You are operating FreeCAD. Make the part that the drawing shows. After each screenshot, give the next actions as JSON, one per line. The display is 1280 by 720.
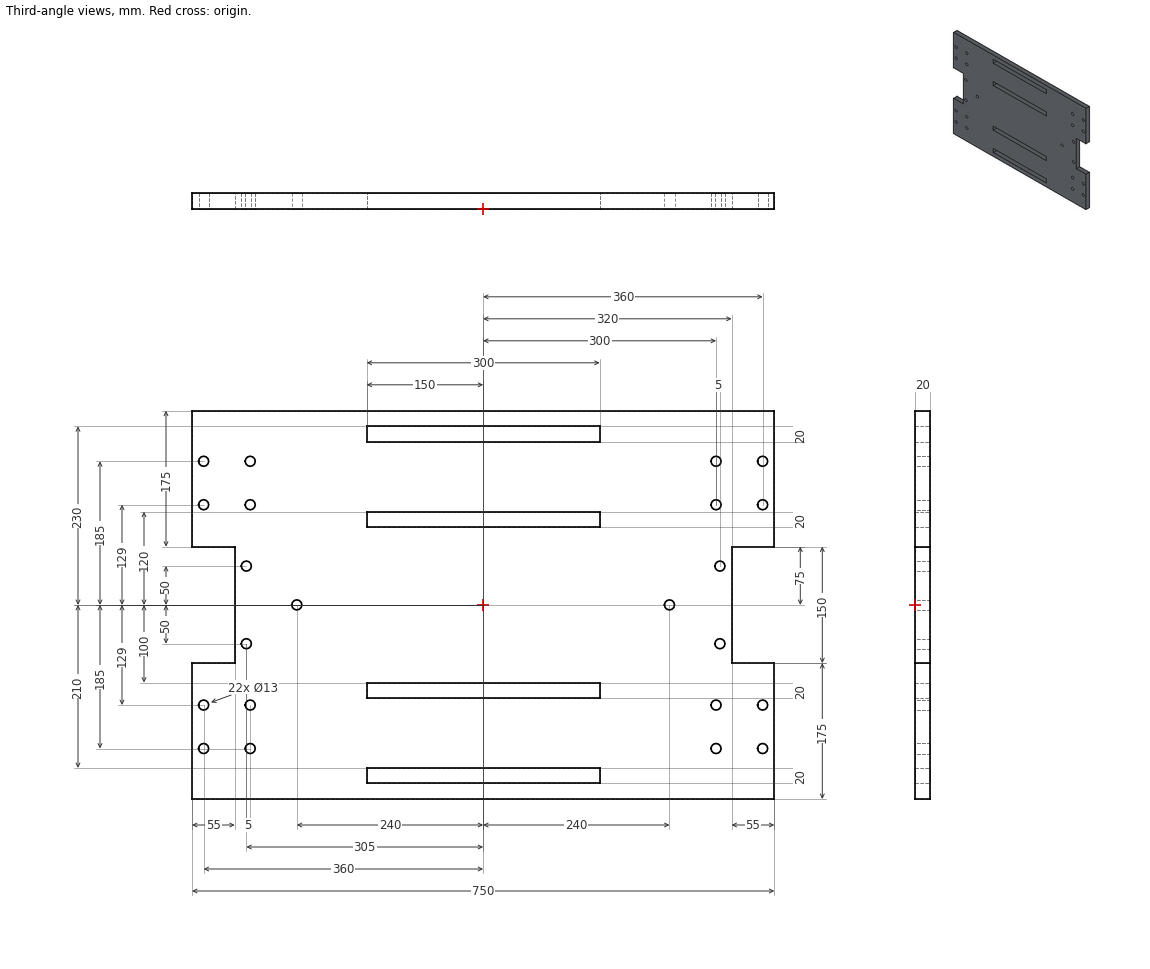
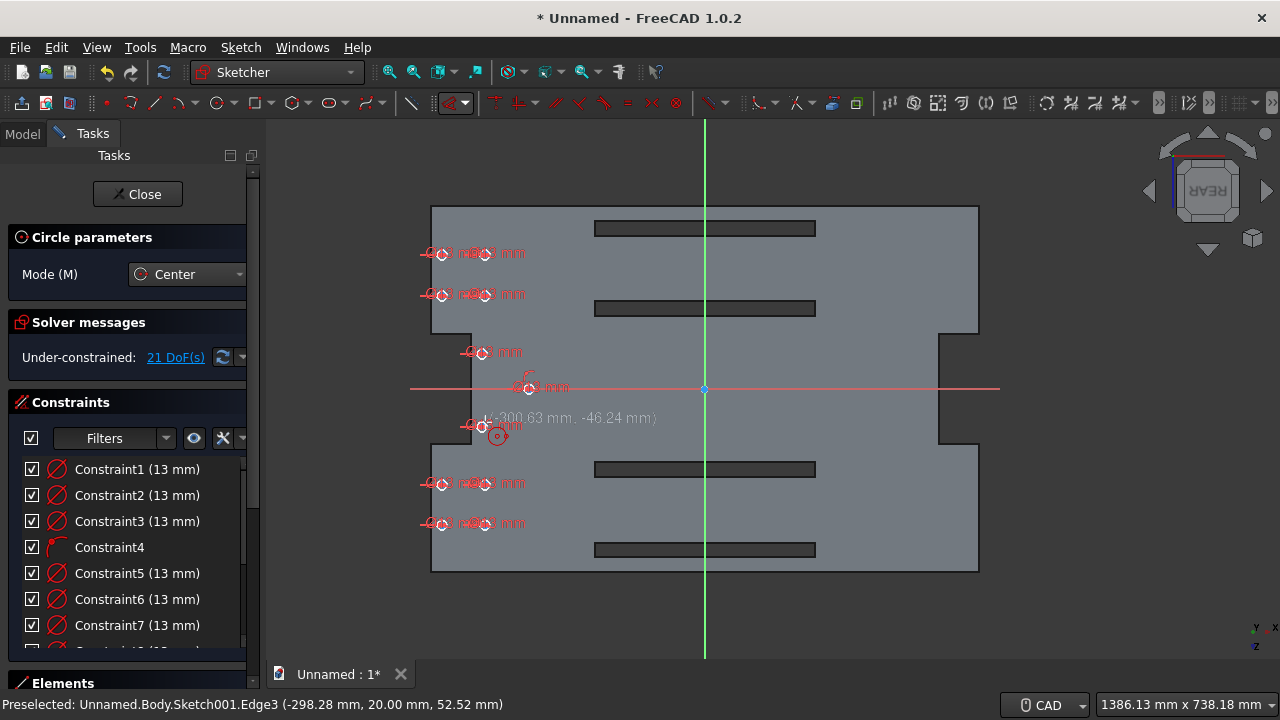
{"action": "scroll", "coordinate": [968, 484], "scroll_direction": "up", "scroll_amount": 8}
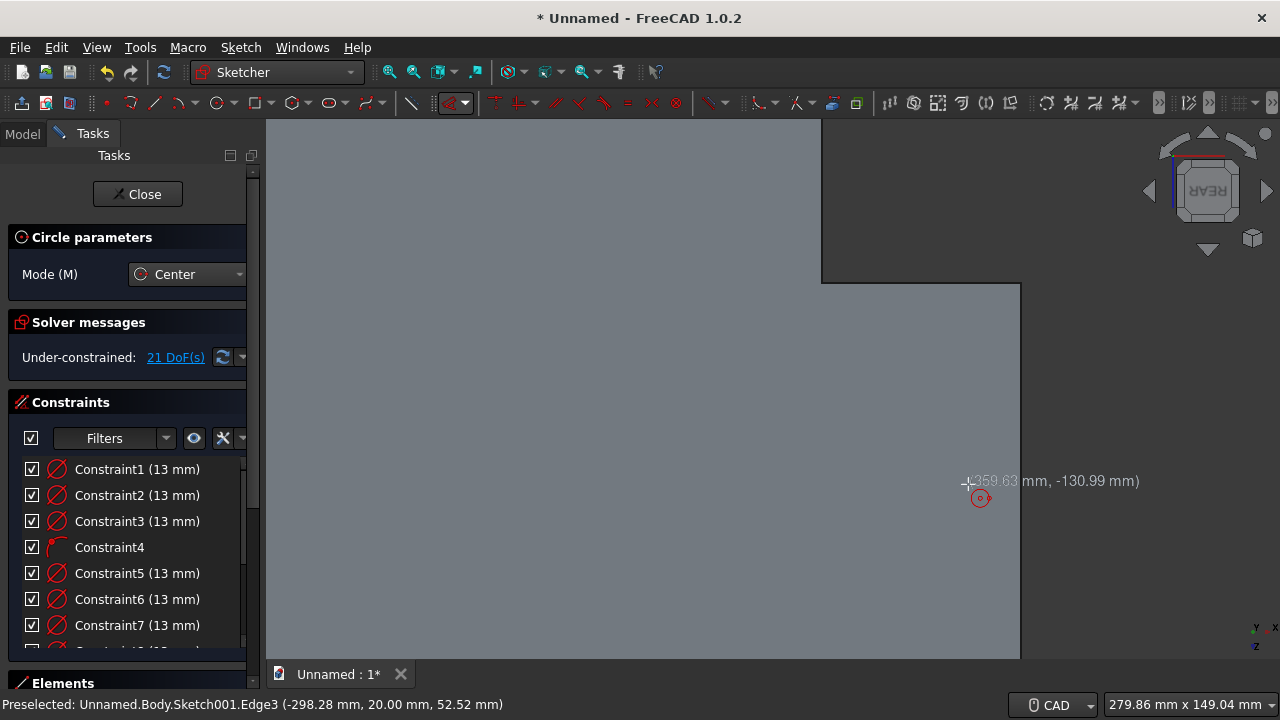
{"action": "scroll", "coordinate": [968, 484], "scroll_direction": "down", "scroll_amount": 8}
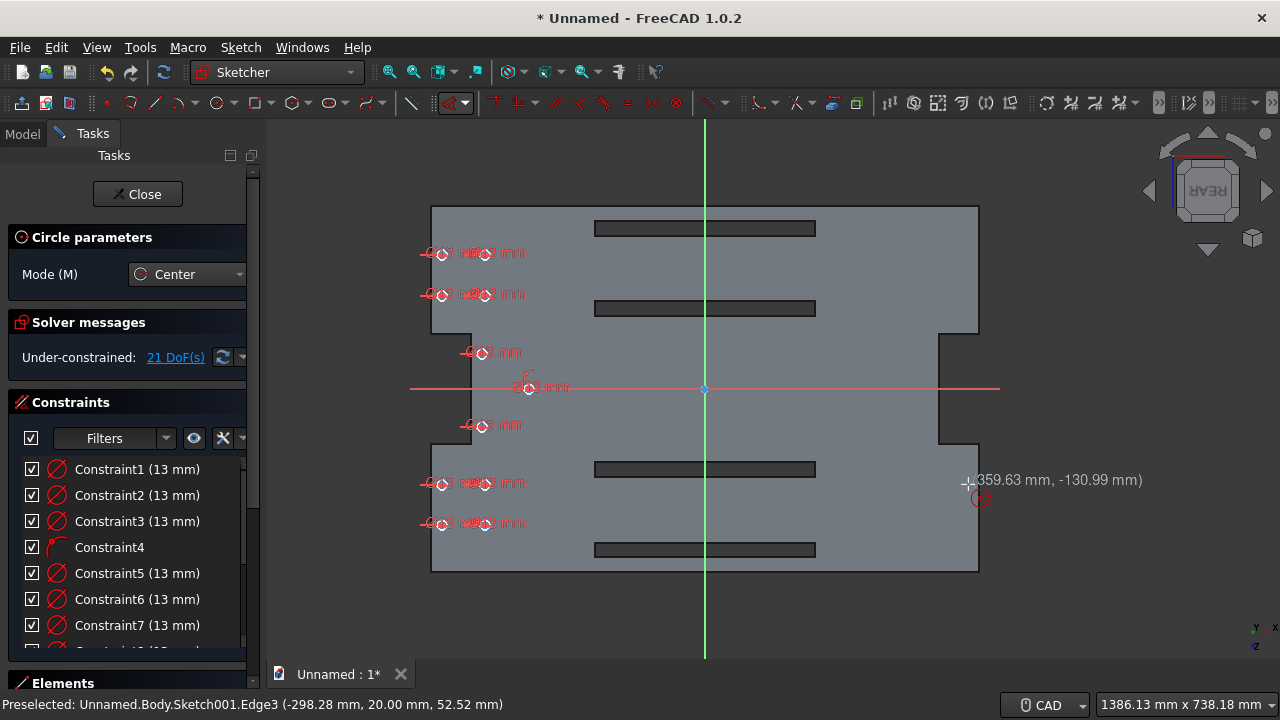
{"action": "left_click", "coordinate": [968, 484]}
{"action": "mouse_move", "coordinate": [972, 480]}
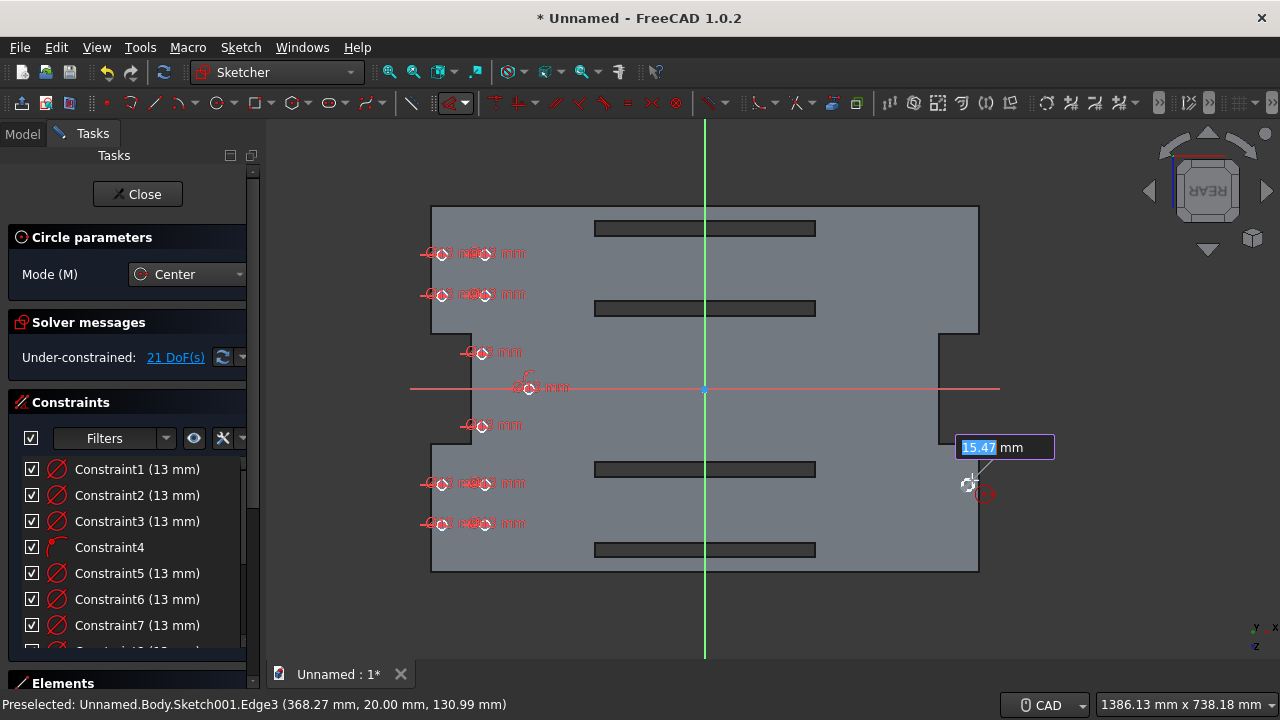
{"action": "type", "text": "13"}
{"action": "key", "text": "Return"}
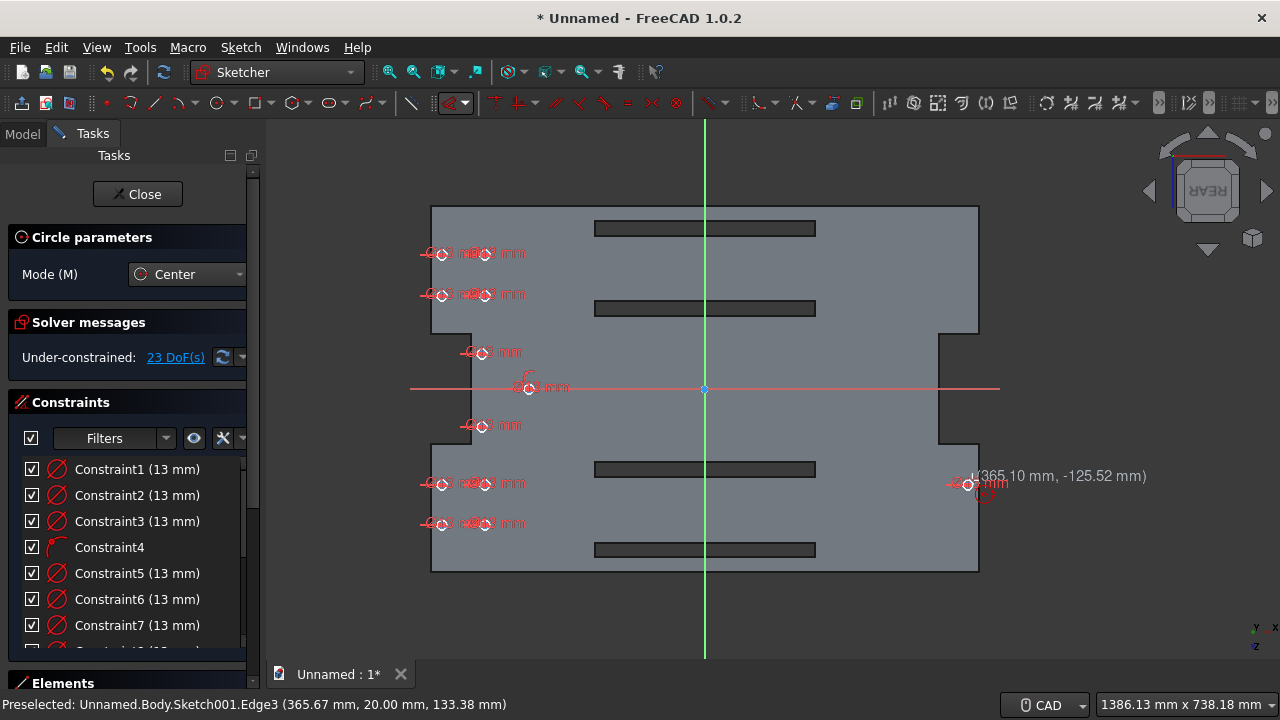
{"action": "scroll", "coordinate": [924, 484], "scroll_direction": "up", "scroll_amount": 8}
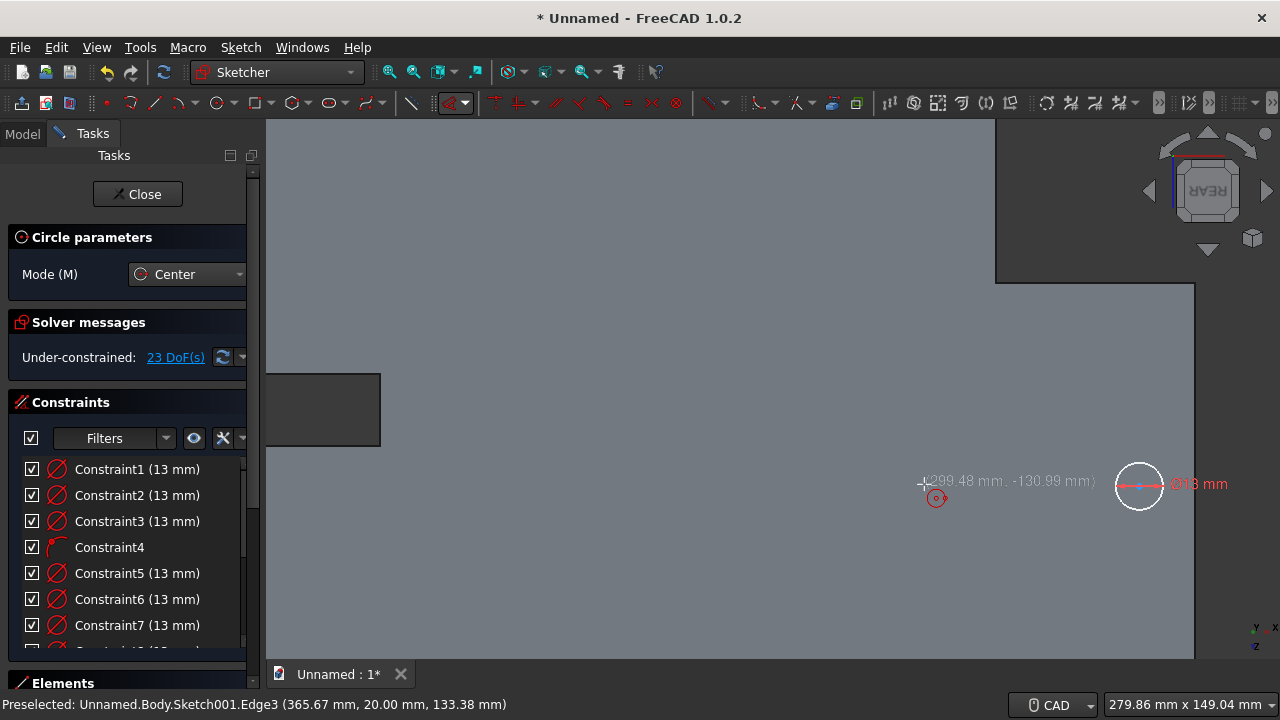
{"action": "scroll", "coordinate": [924, 484], "scroll_direction": "down", "scroll_amount": 8}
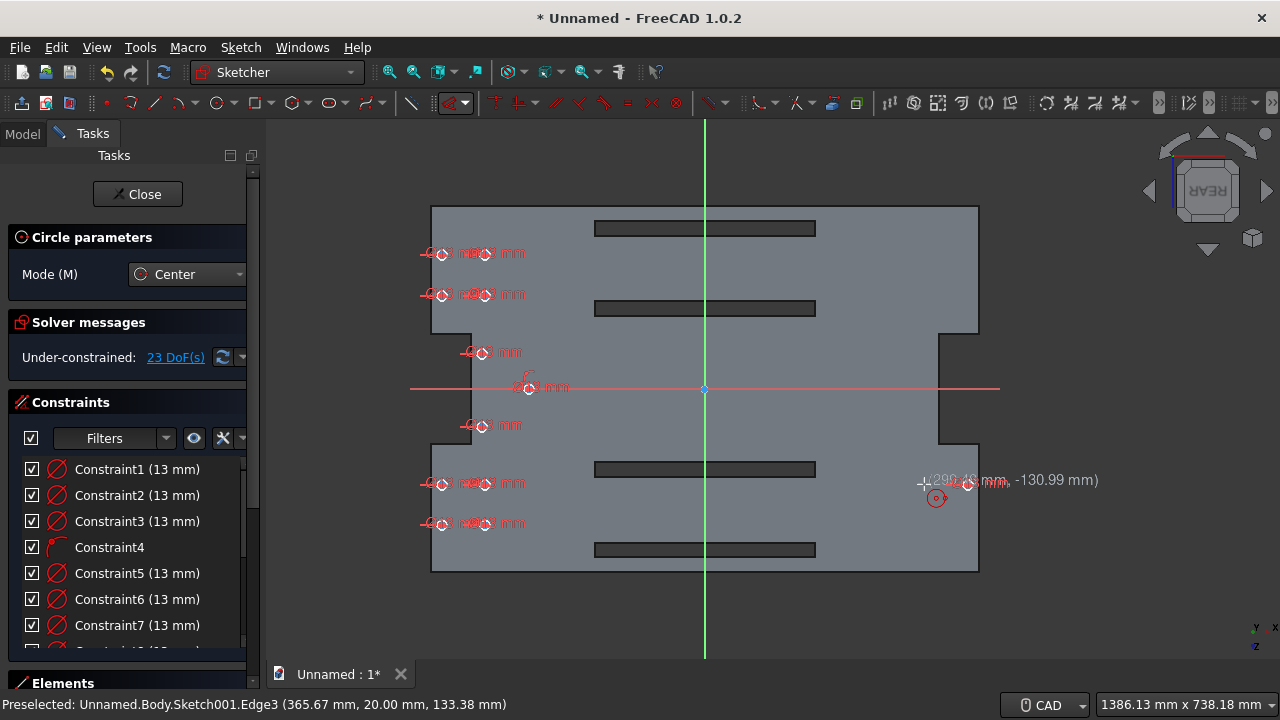
{"action": "left_click", "coordinate": [924, 484]}
{"action": "mouse_move", "coordinate": [928, 480]}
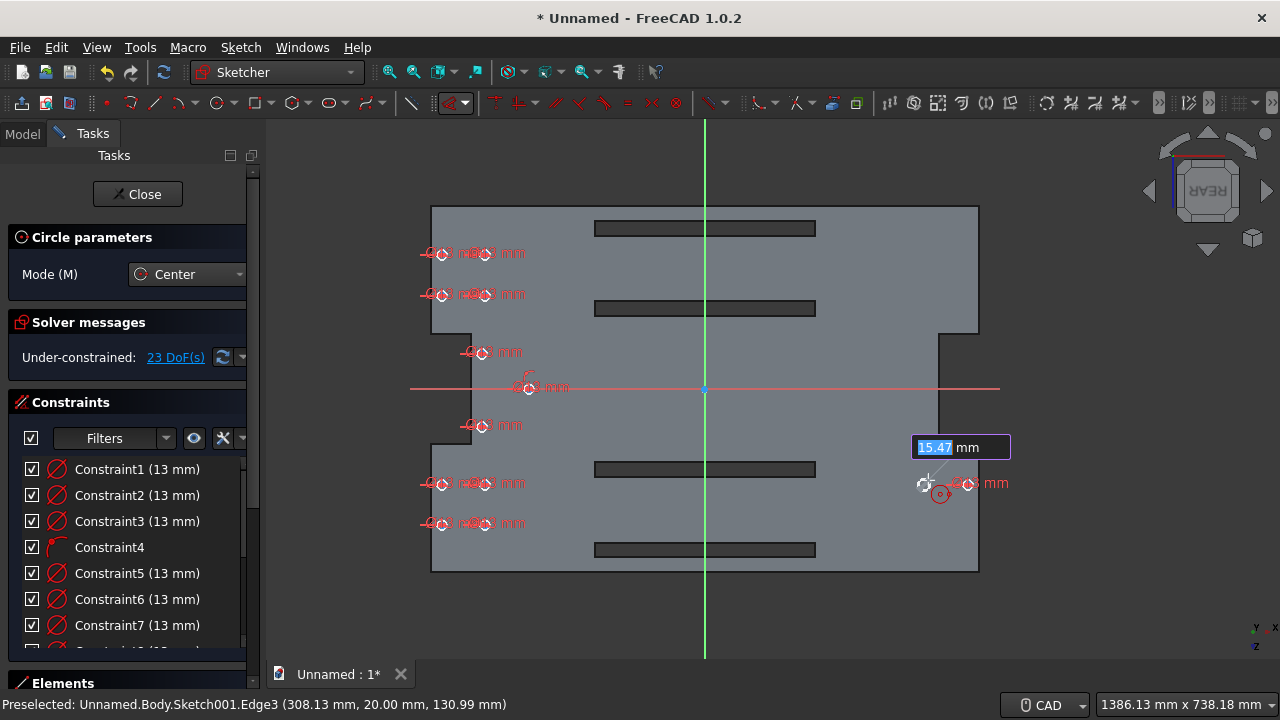
{"action": "type", "text": "13"}
{"action": "key", "text": "Return"}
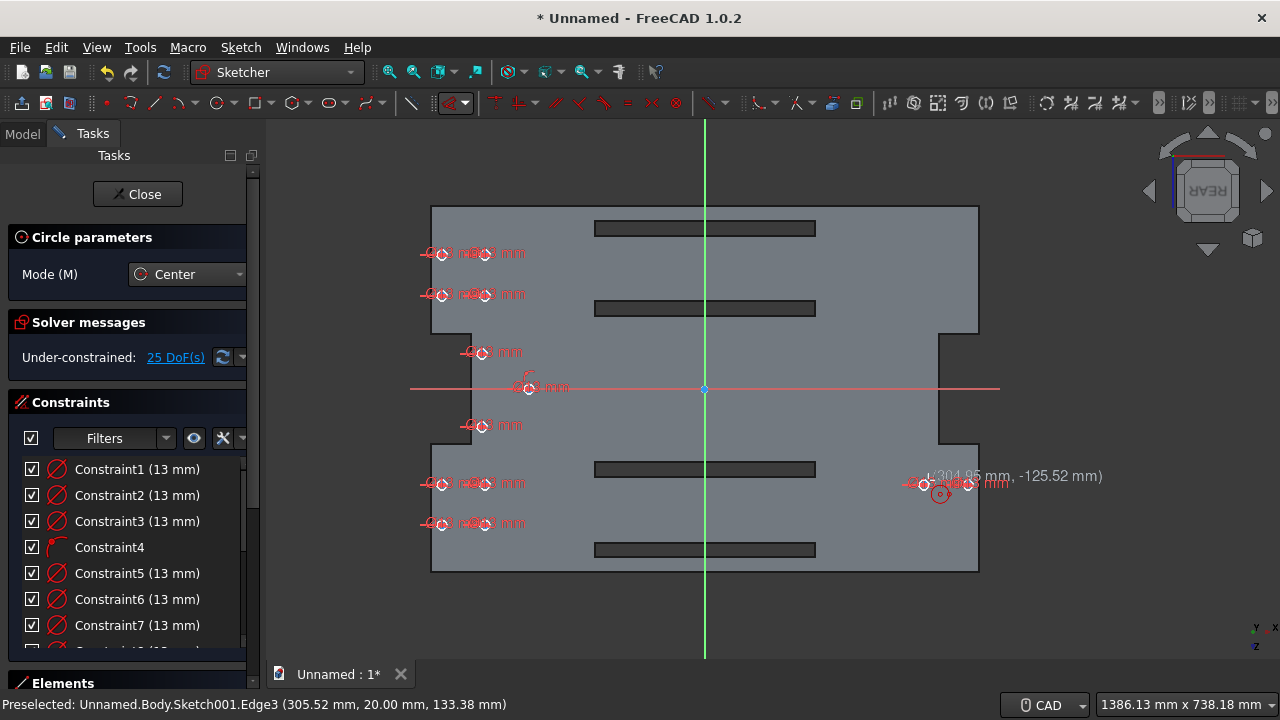
{"action": "scroll", "coordinate": [968, 525], "scroll_direction": "up", "scroll_amount": 8}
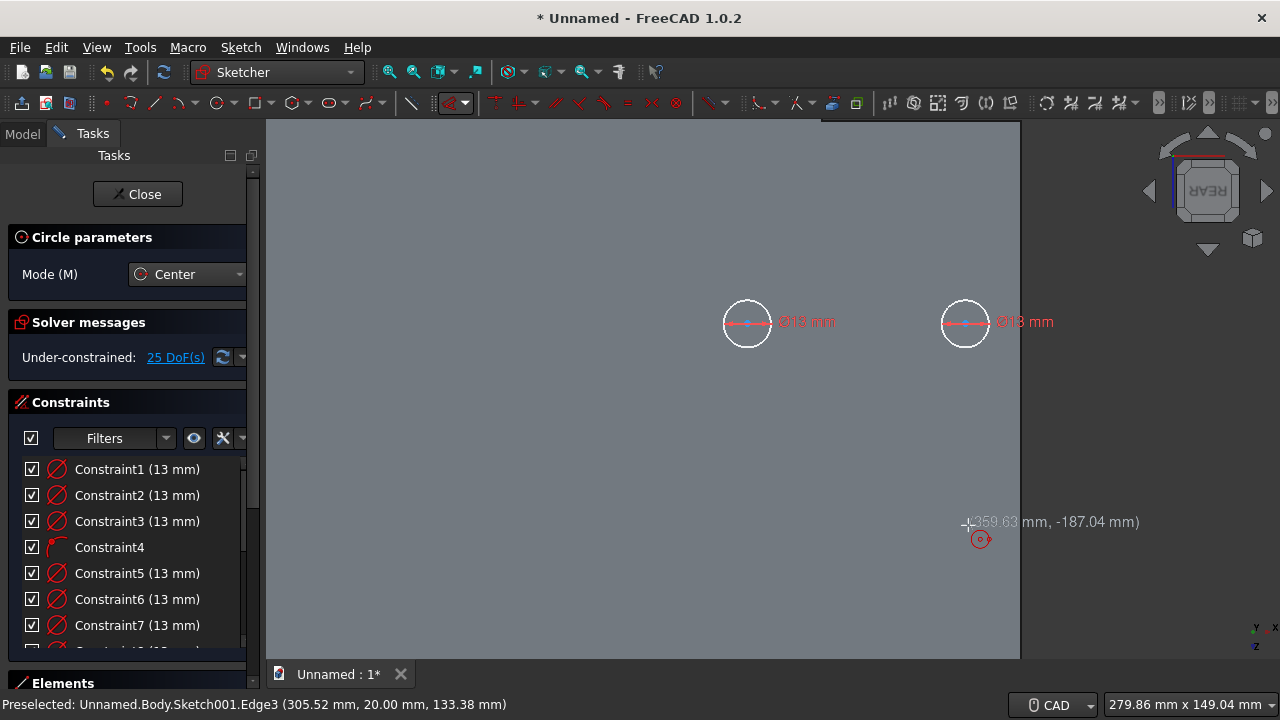
{"action": "scroll", "coordinate": [968, 526], "scroll_direction": "down", "scroll_amount": 8}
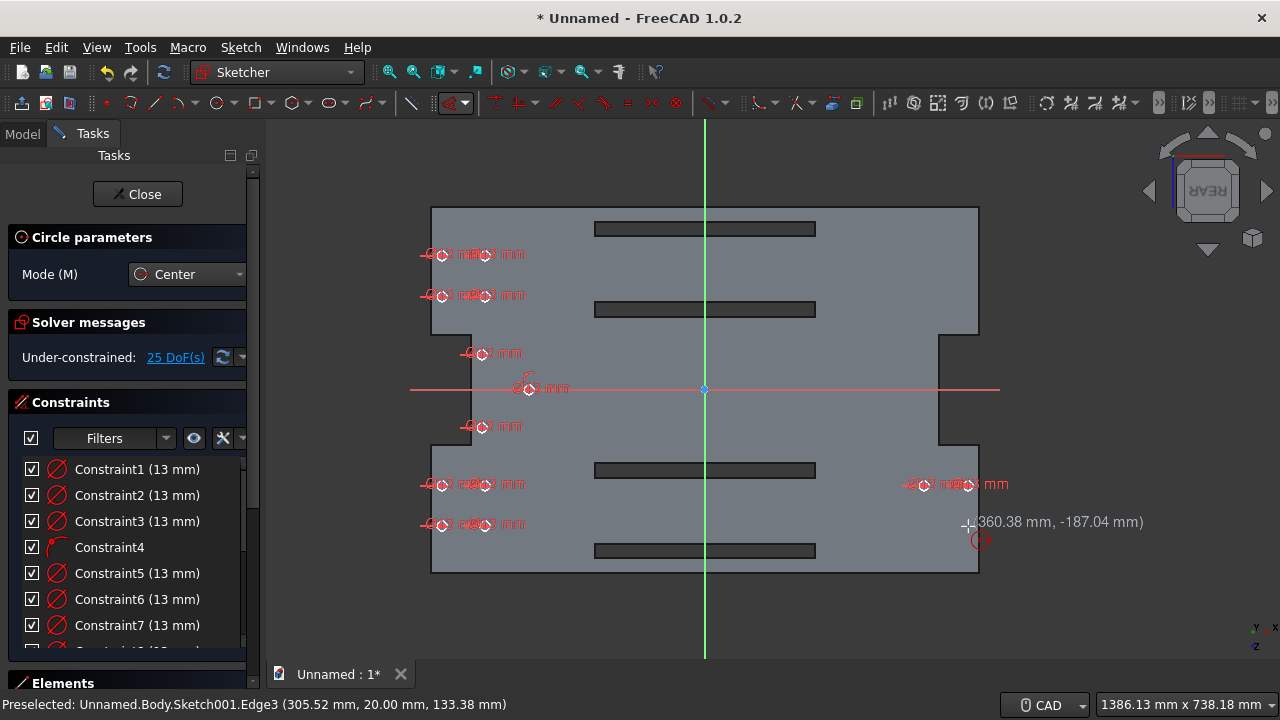
{"action": "left_click", "coordinate": [968, 525]}
{"action": "mouse_move", "coordinate": [972, 522]}